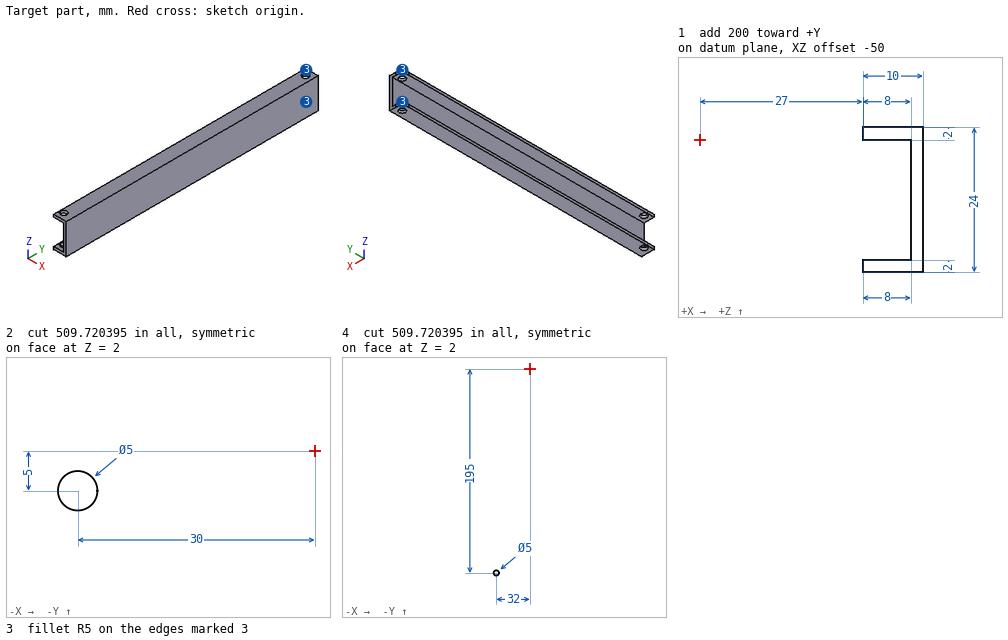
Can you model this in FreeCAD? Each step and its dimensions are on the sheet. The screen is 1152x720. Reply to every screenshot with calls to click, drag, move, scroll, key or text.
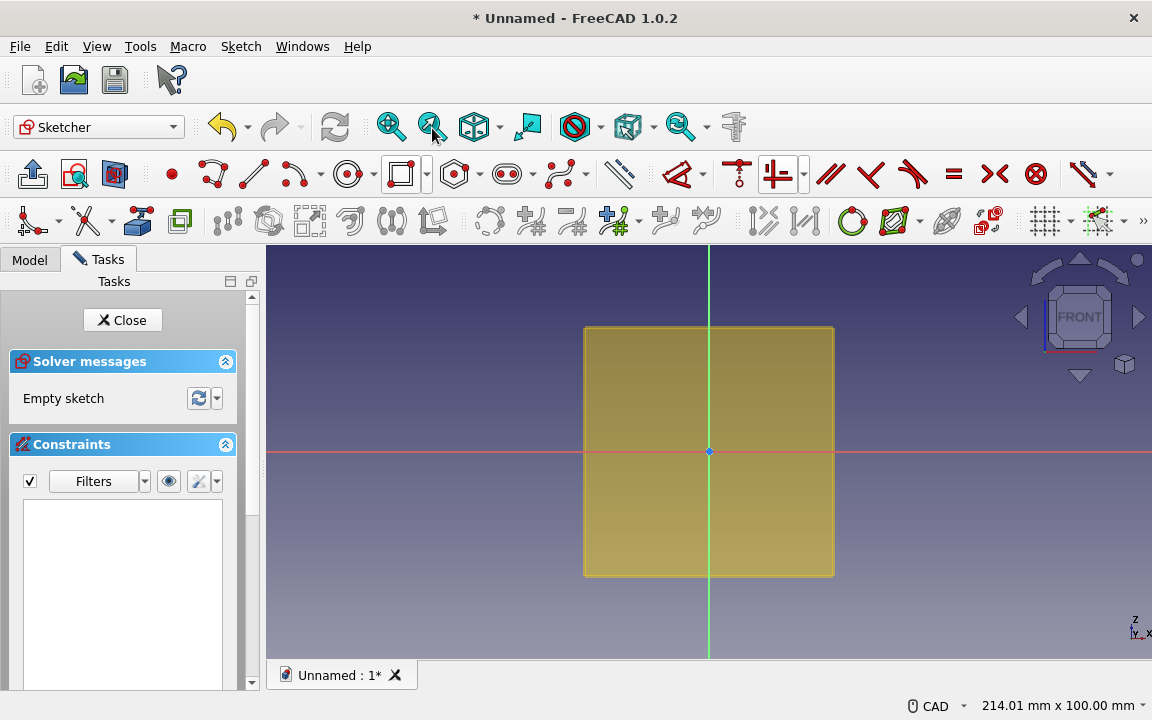
scroll(870, 517, up, 5)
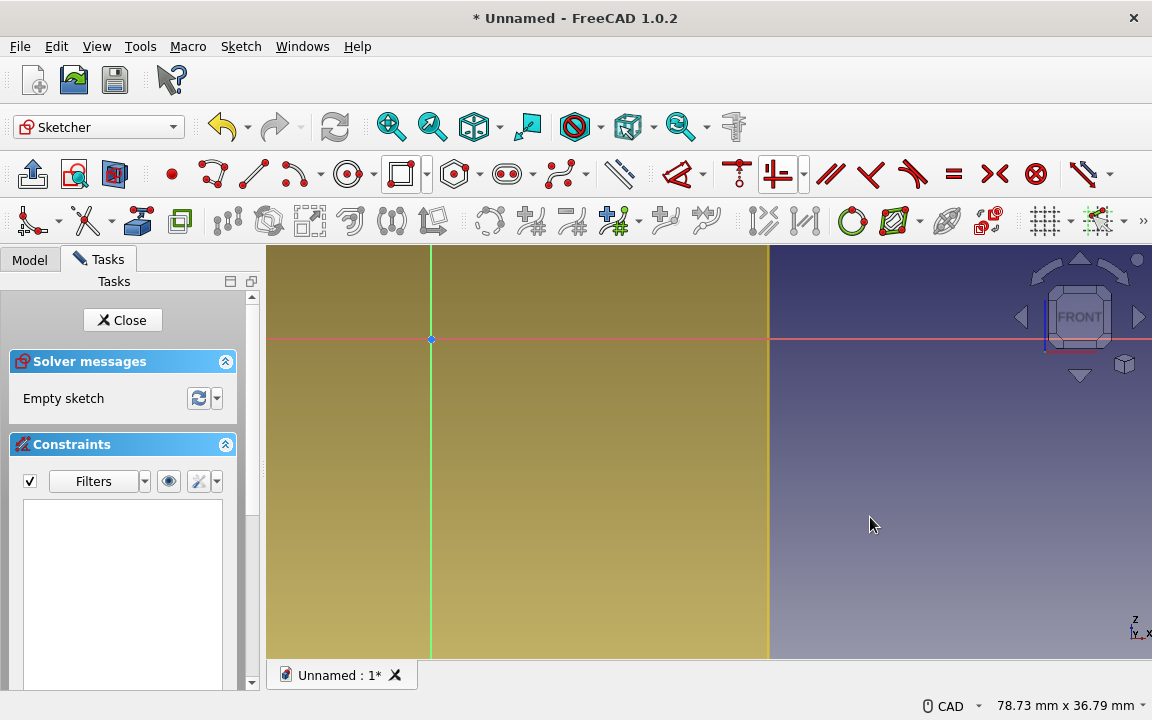
click(213, 174)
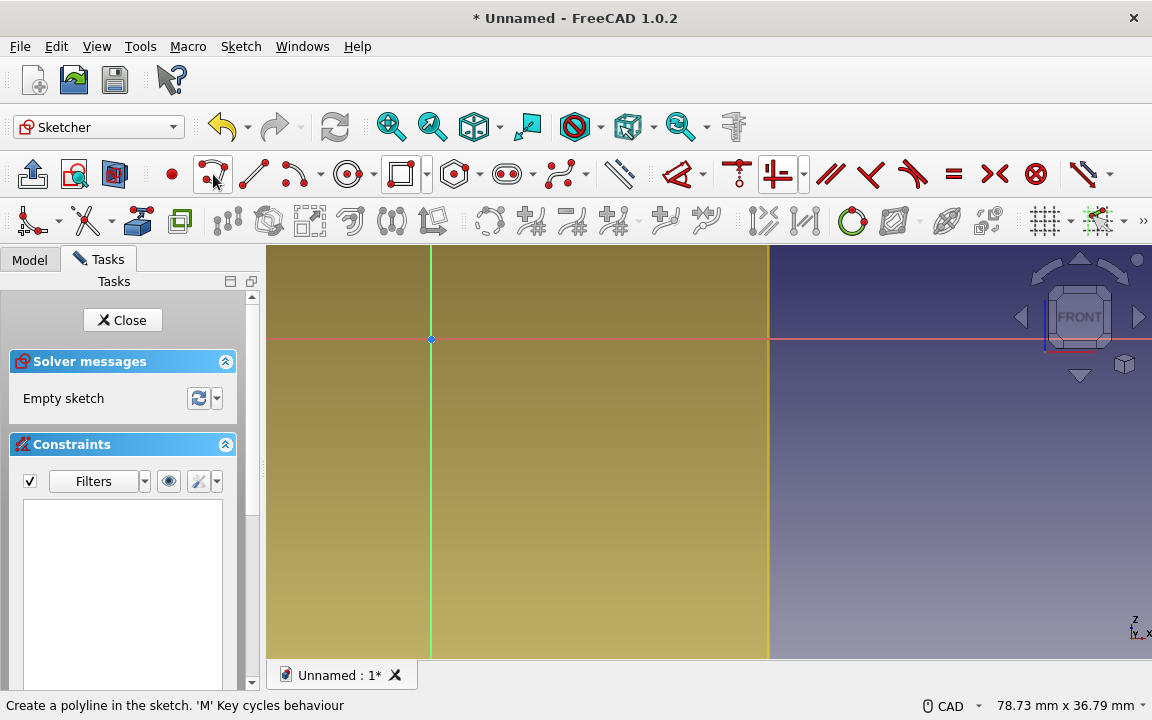
click(735, 339)
click(735, 317)
click(848, 317)
click(848, 587)
click(735, 587)
click(735, 564)
click(825, 564)
click(825, 348)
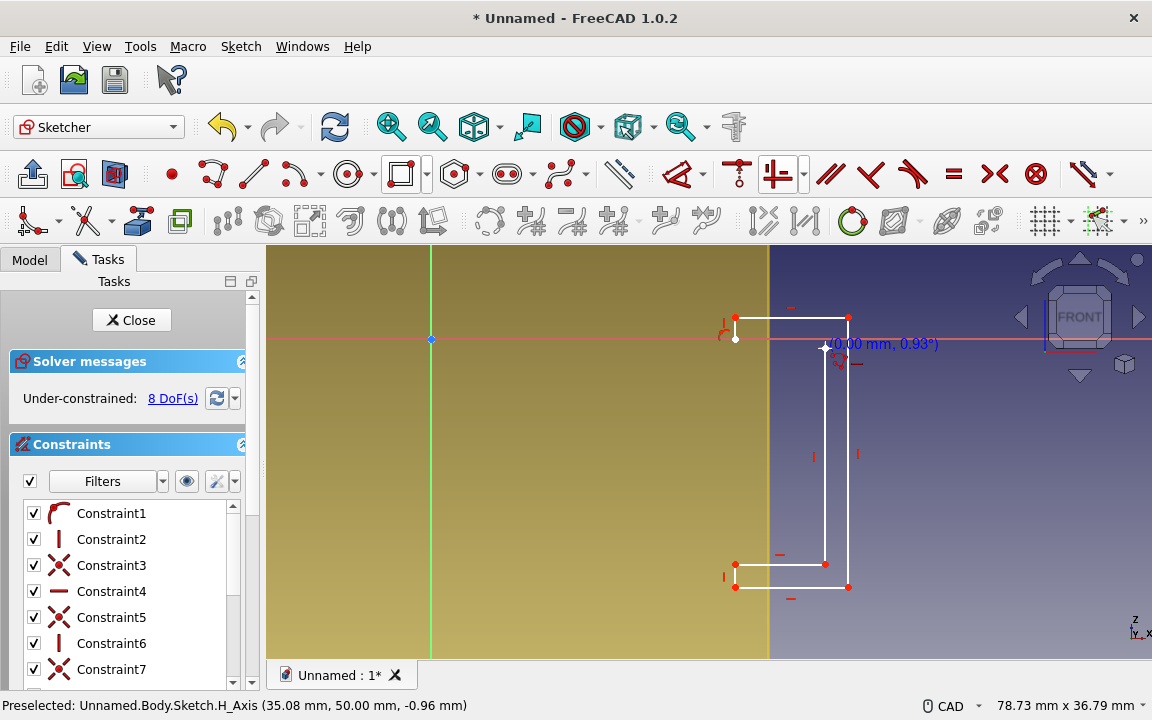
scroll(735, 339, up, 2)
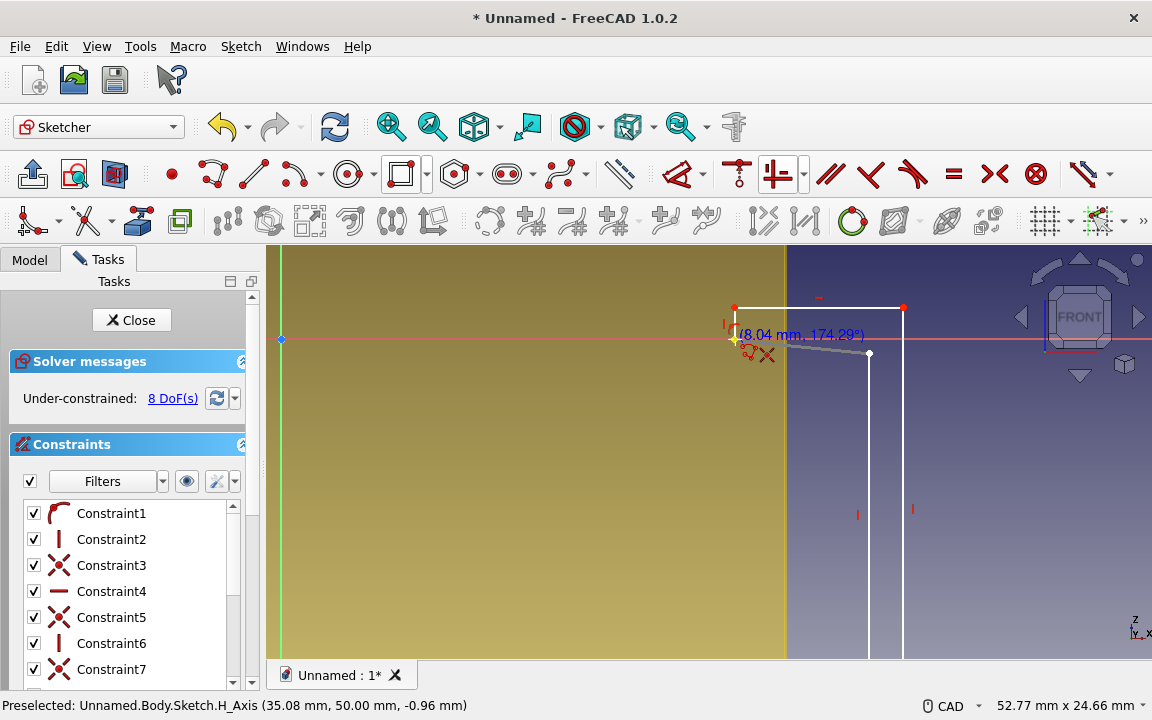
click(735, 339)
key(Escape)
key(Escape)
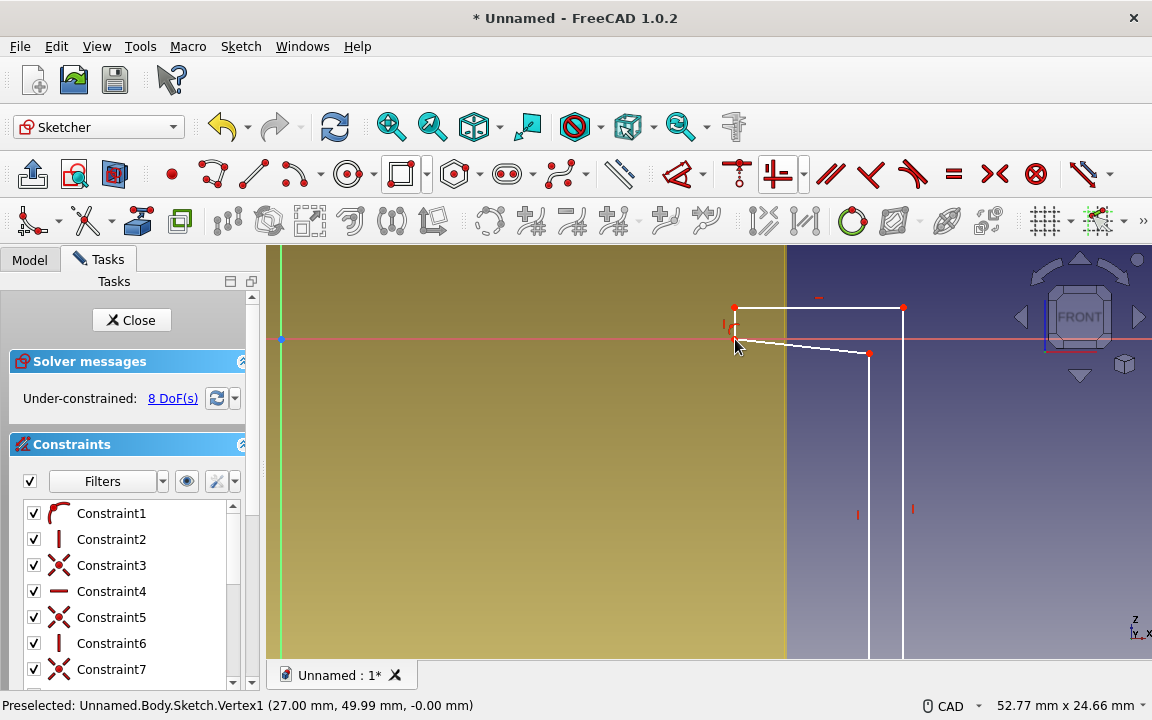
scroll(829, 349, up, 2)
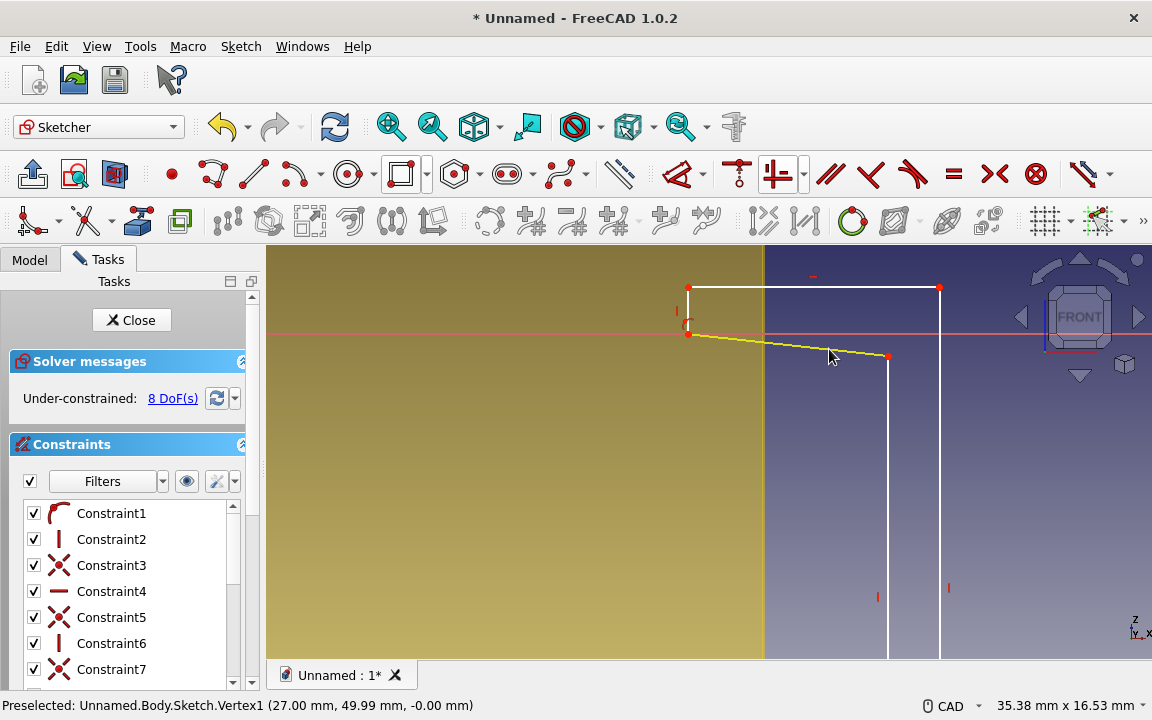
click(828, 349)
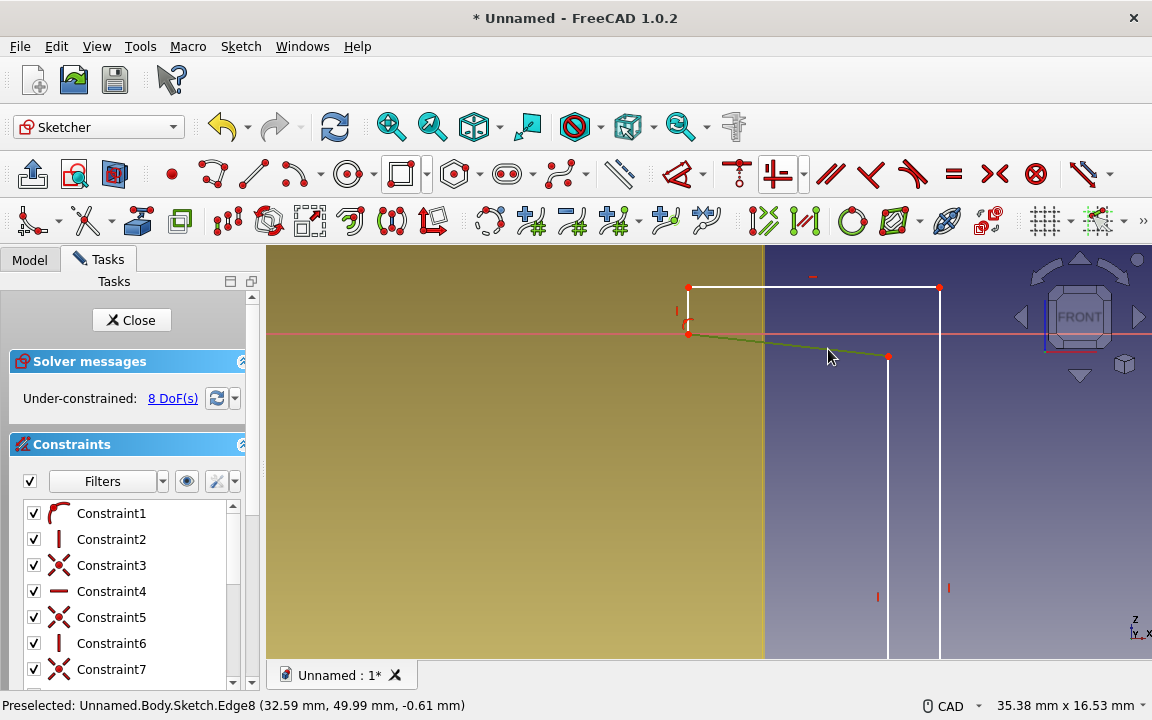
key(h)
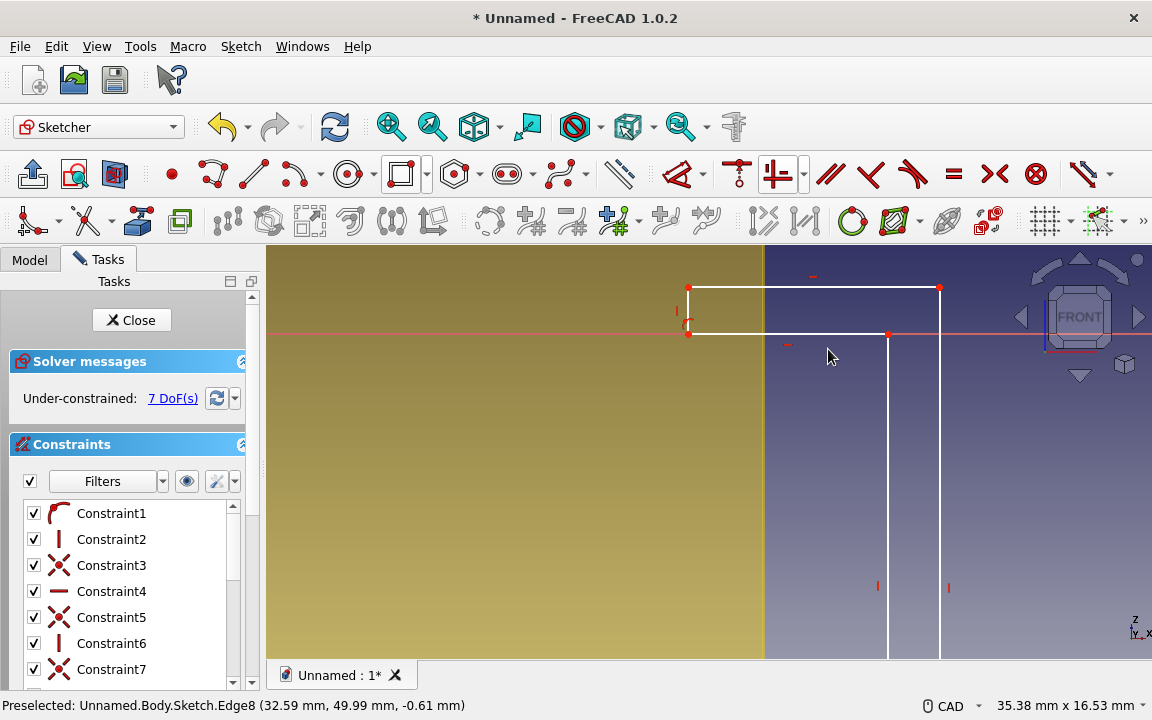
click(676, 174)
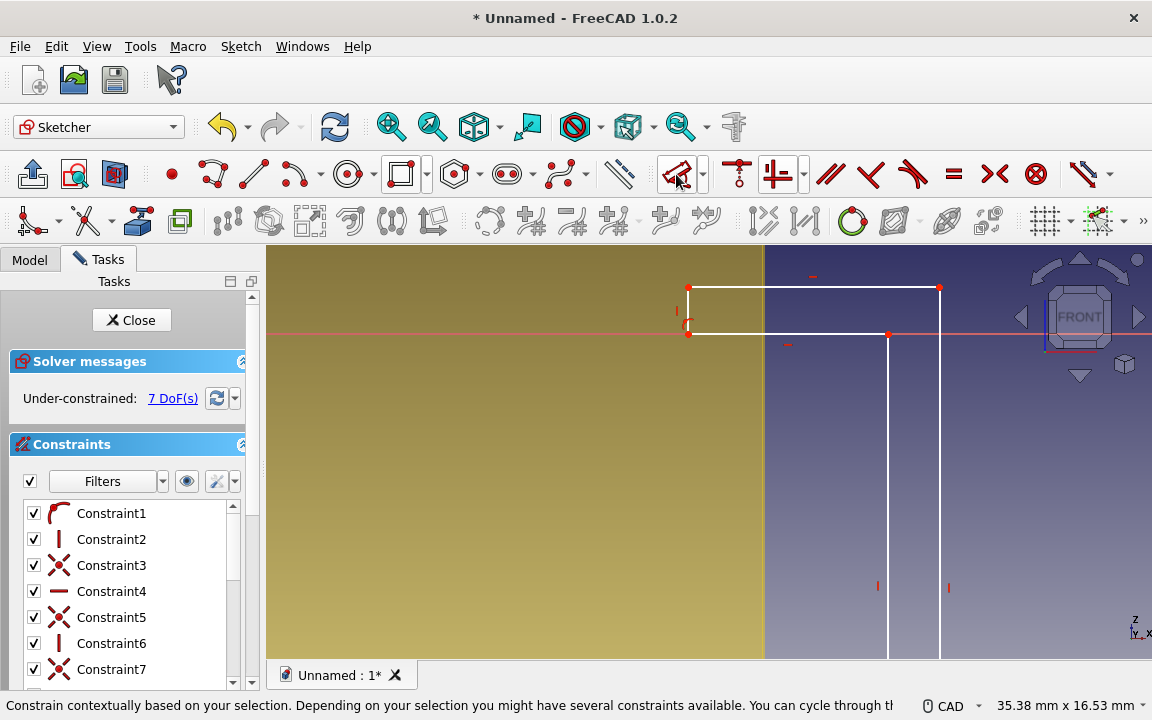
click(688, 320)
click(722, 311)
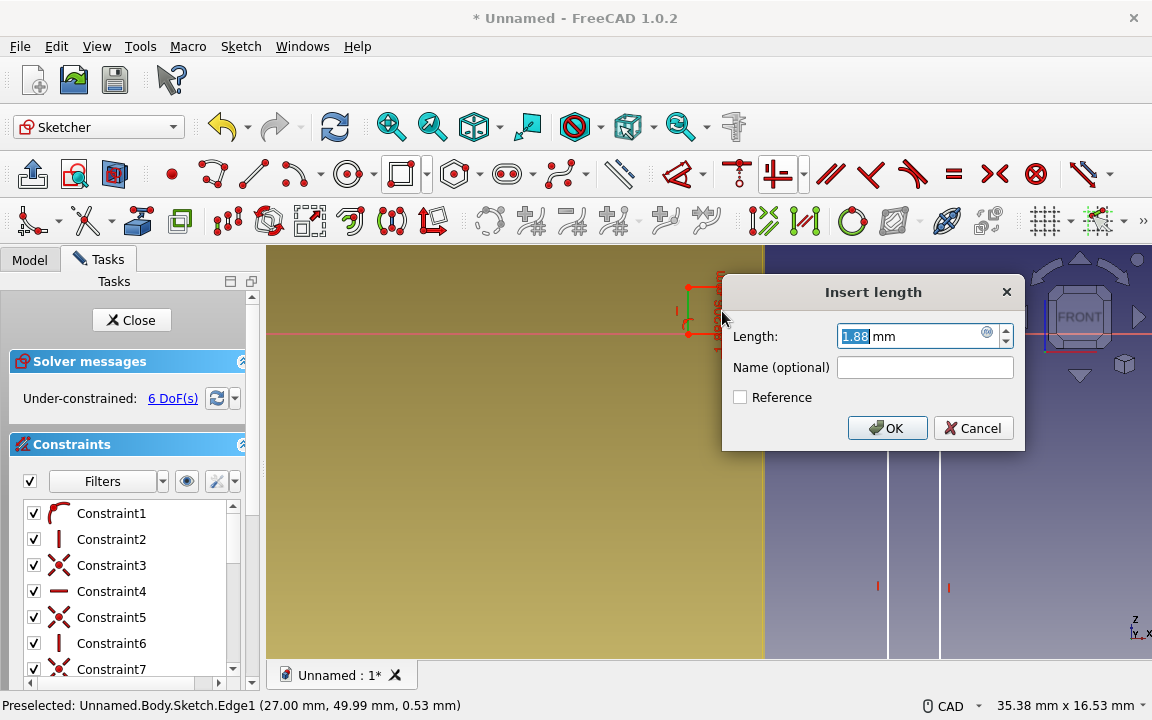
text(2)
key(Return)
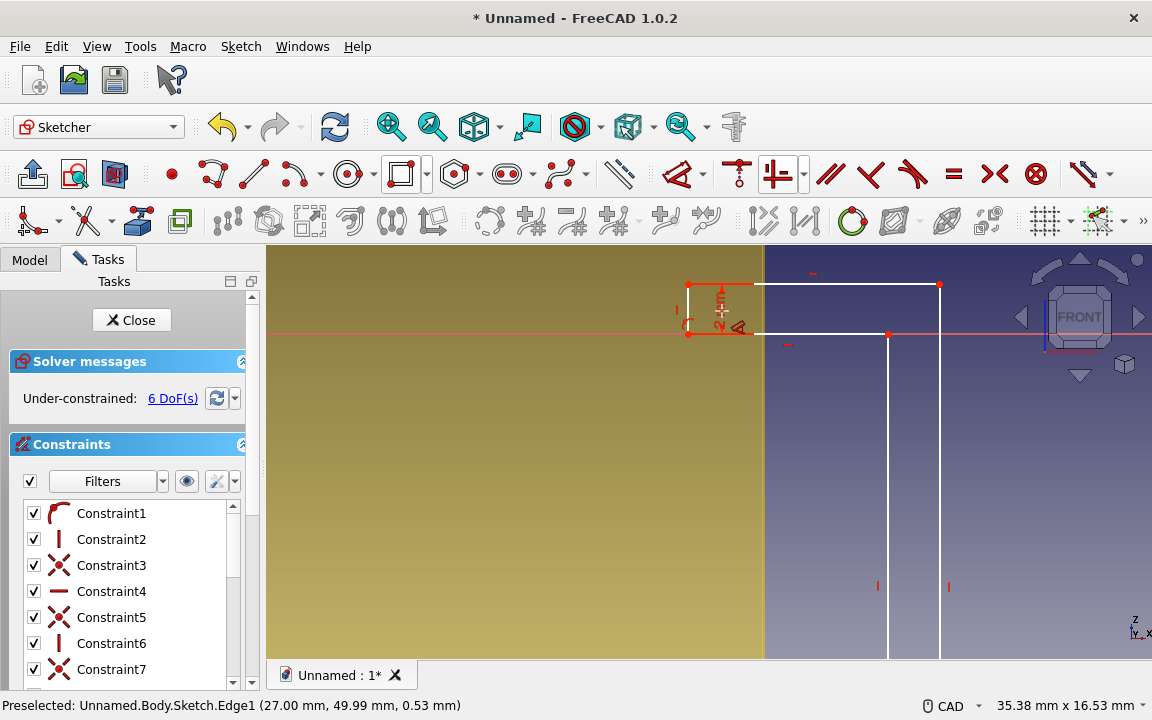
scroll(775, 344, down, 4)